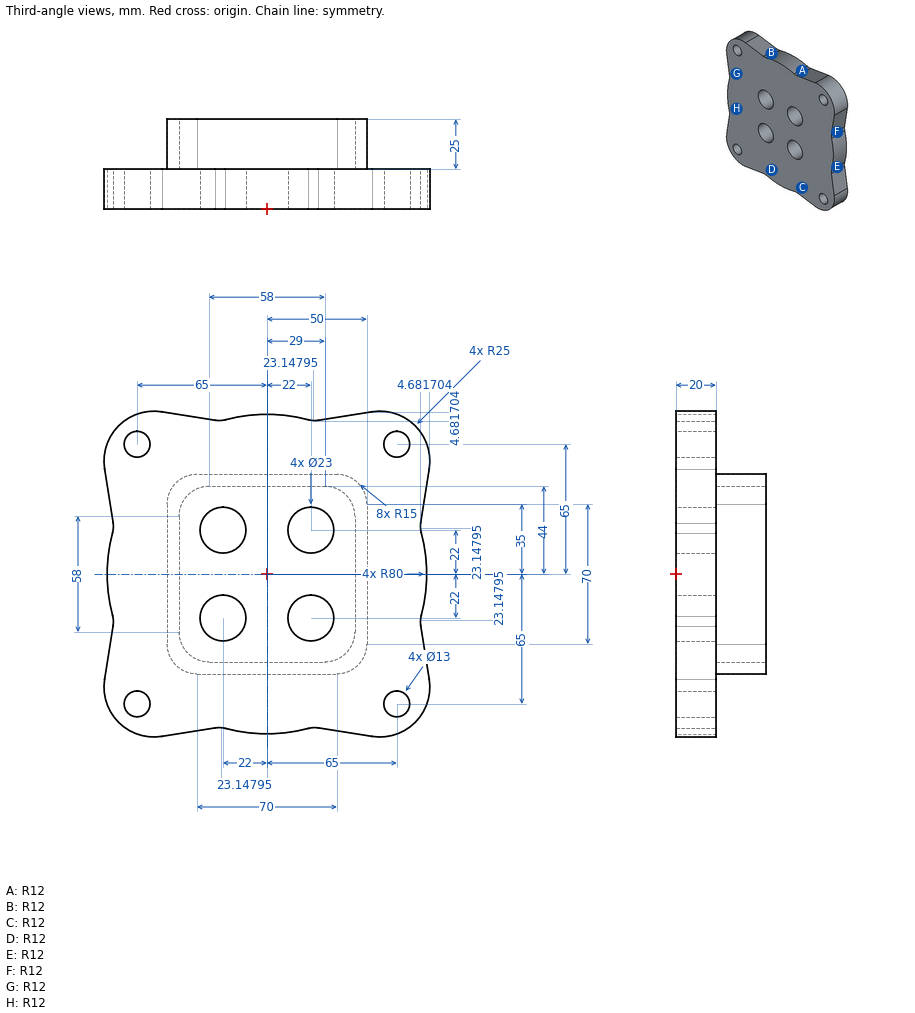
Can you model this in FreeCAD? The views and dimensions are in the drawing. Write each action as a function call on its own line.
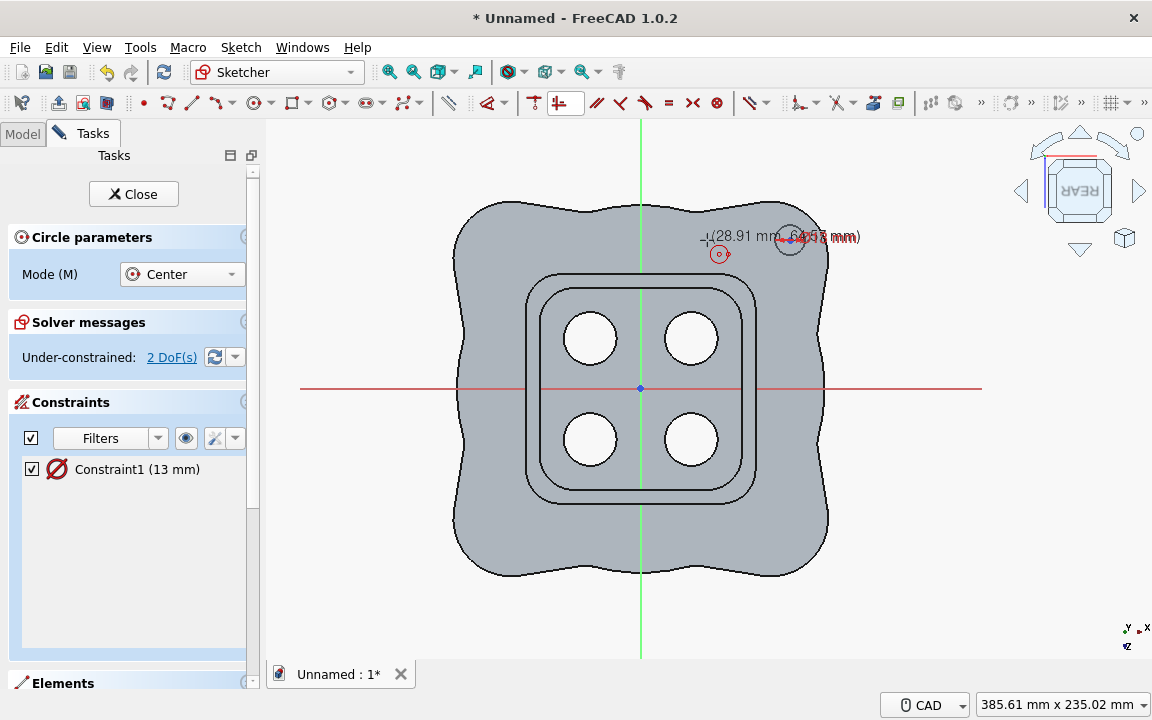
scroll(790, 538, up, 3)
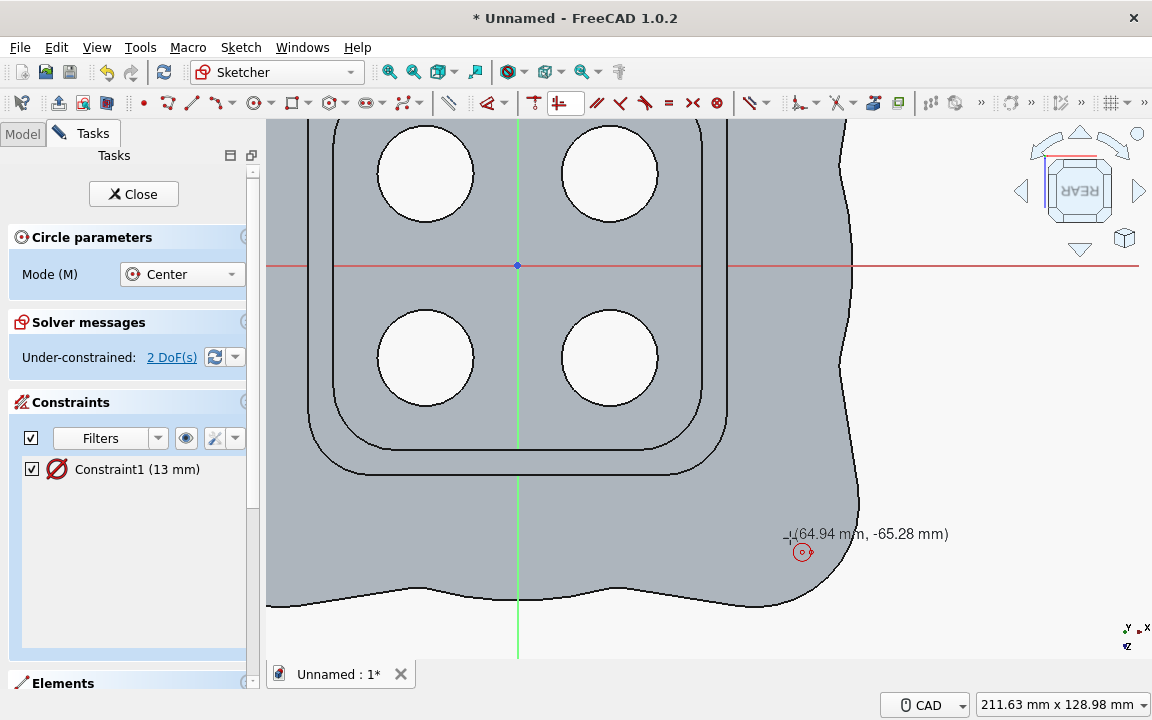
click(790, 538)
move(809, 519)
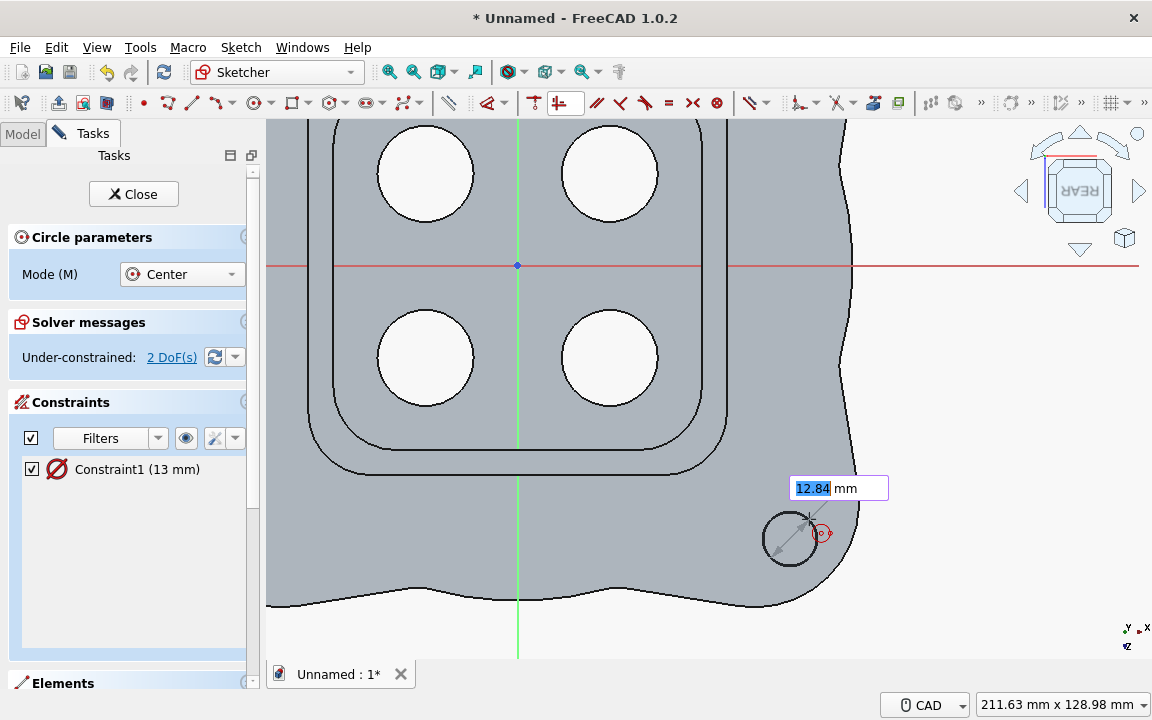
text(13)
key(Return)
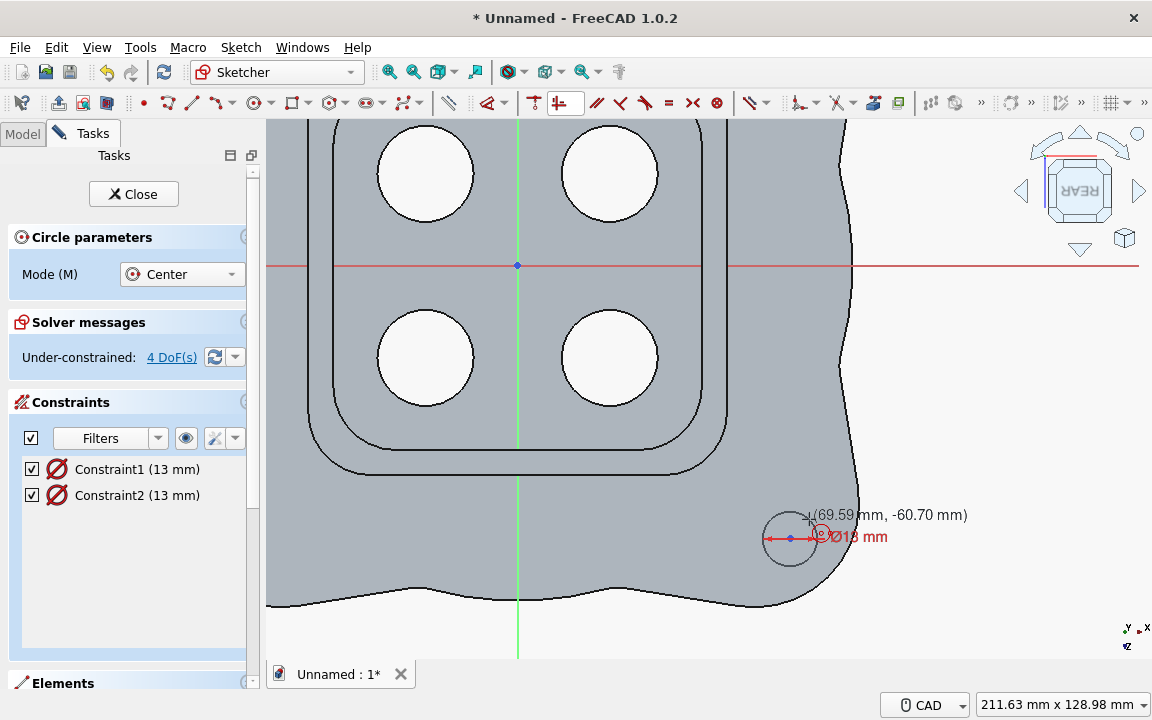
scroll(790, 539, down, 3)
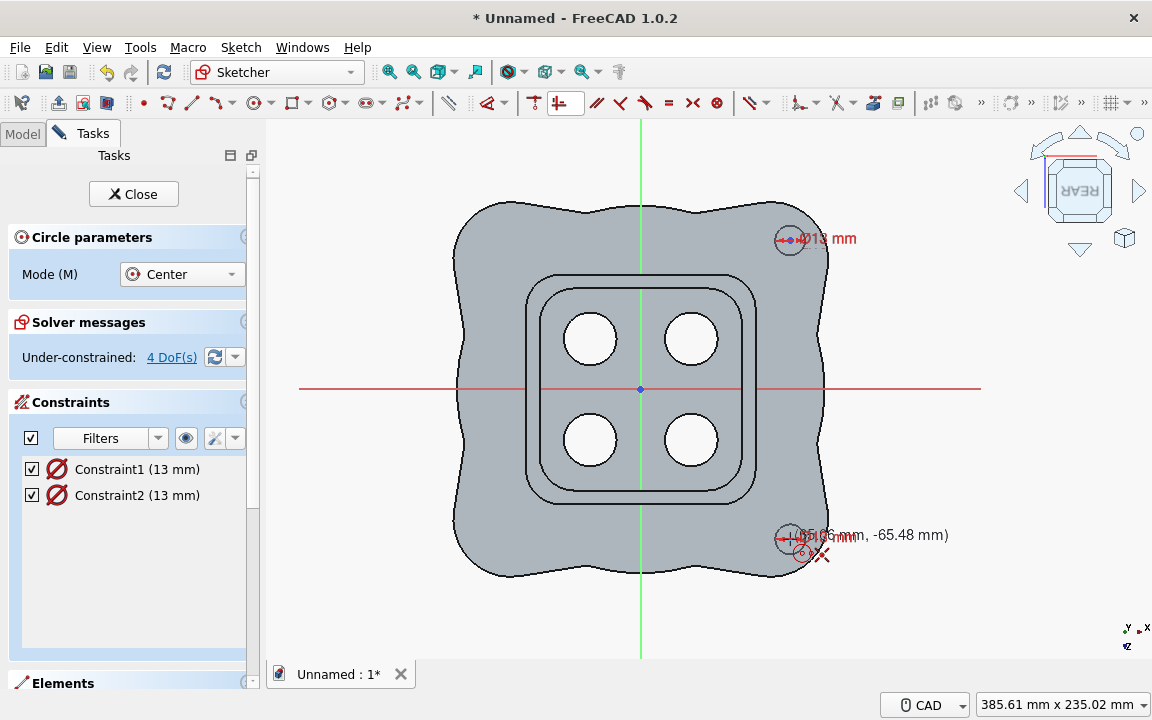
scroll(491, 539, up, 3)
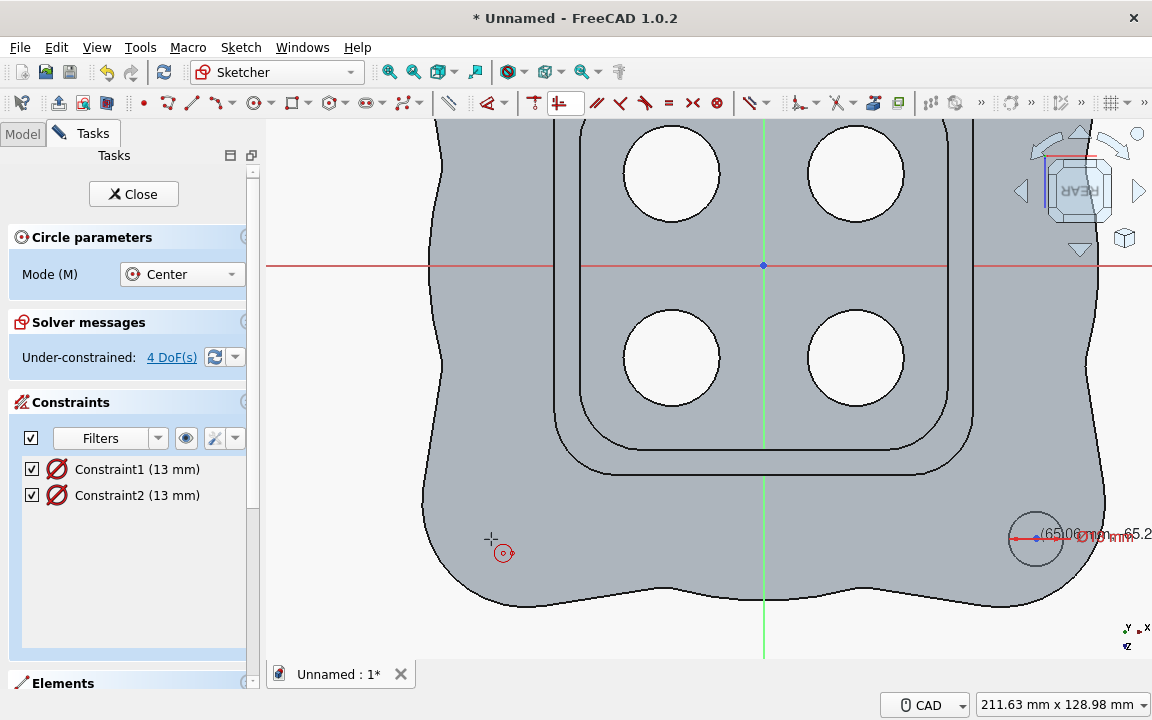
click(492, 538)
move(511, 519)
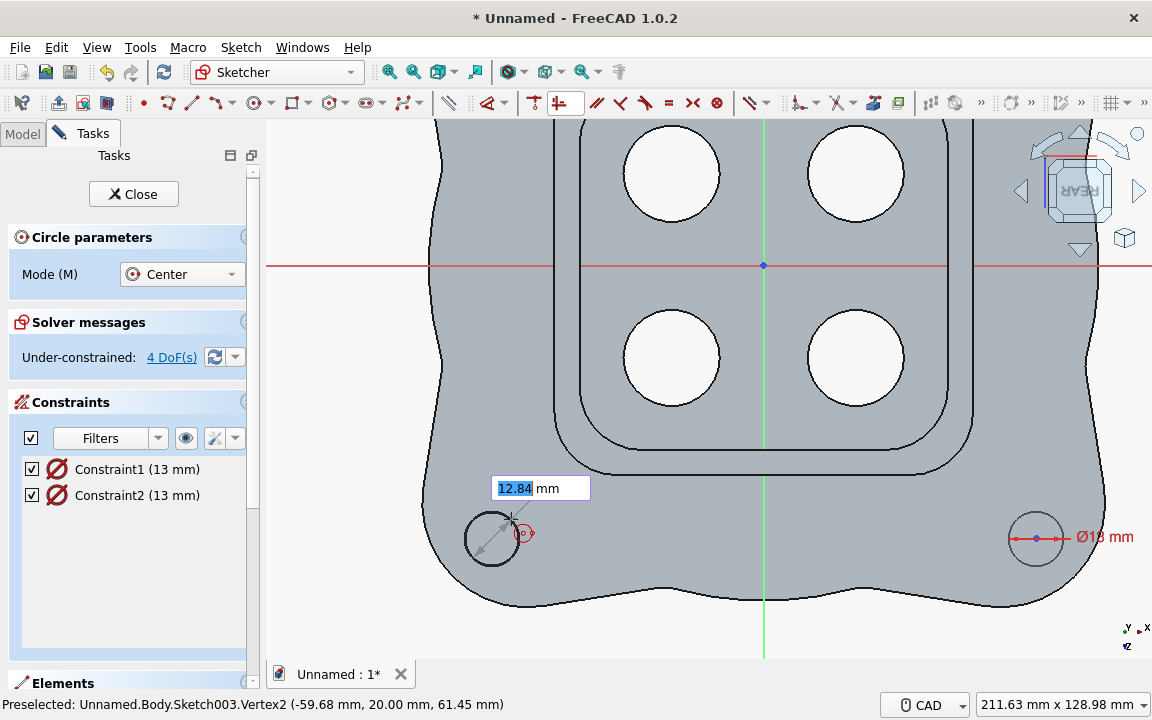
text(13)
key(Return)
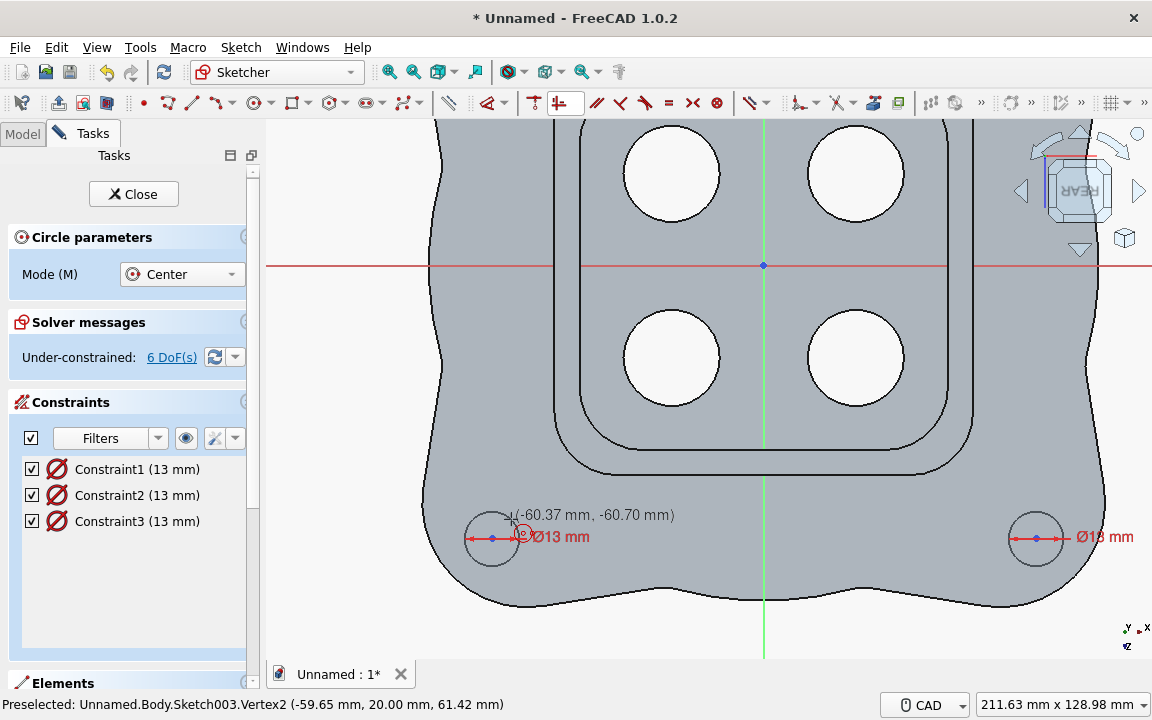
scroll(491, 539, down, 3)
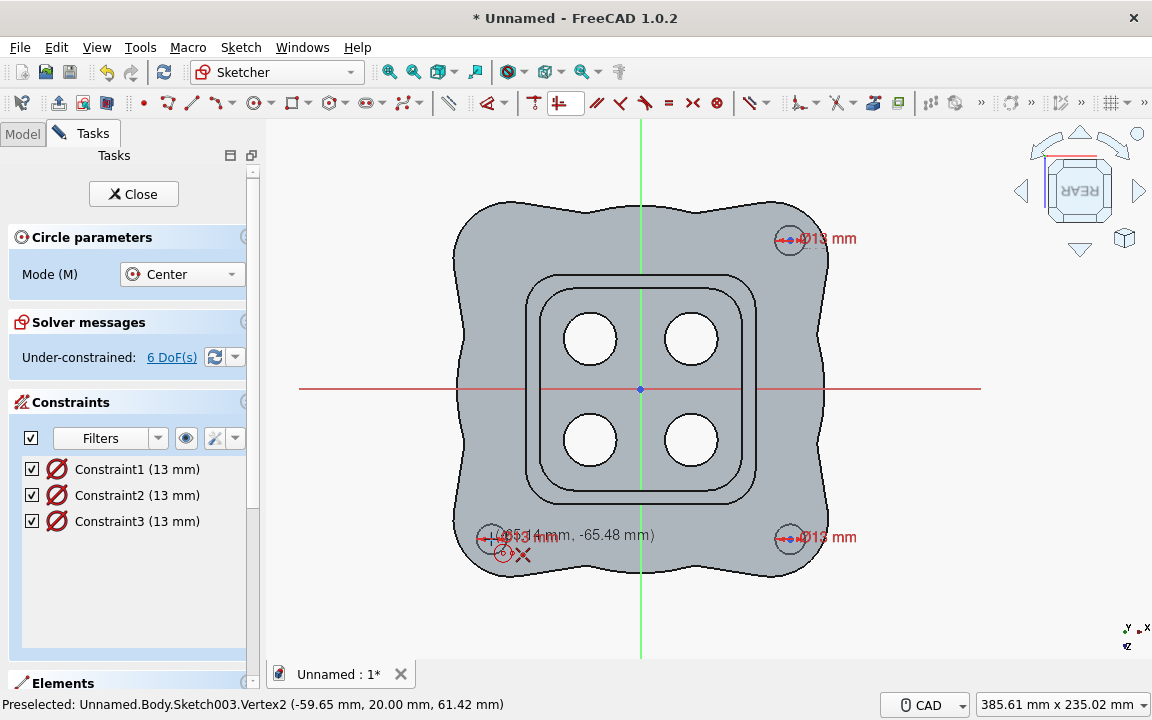
scroll(491, 240, up, 3)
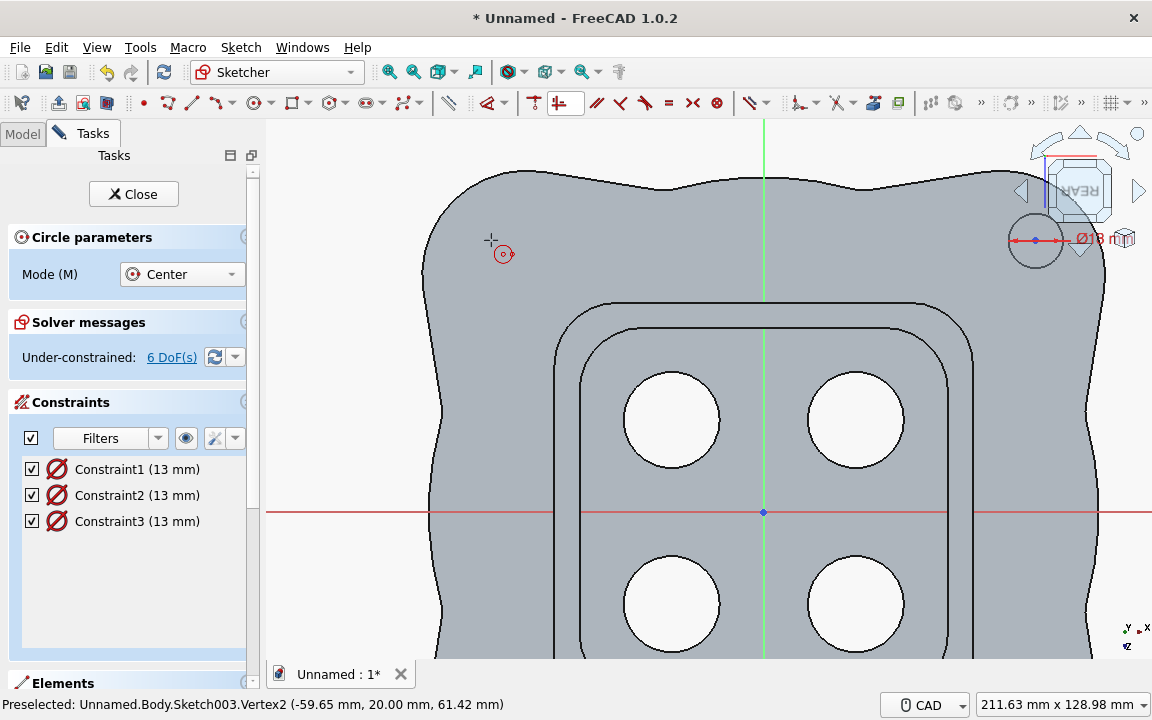
click(492, 240)
move(511, 221)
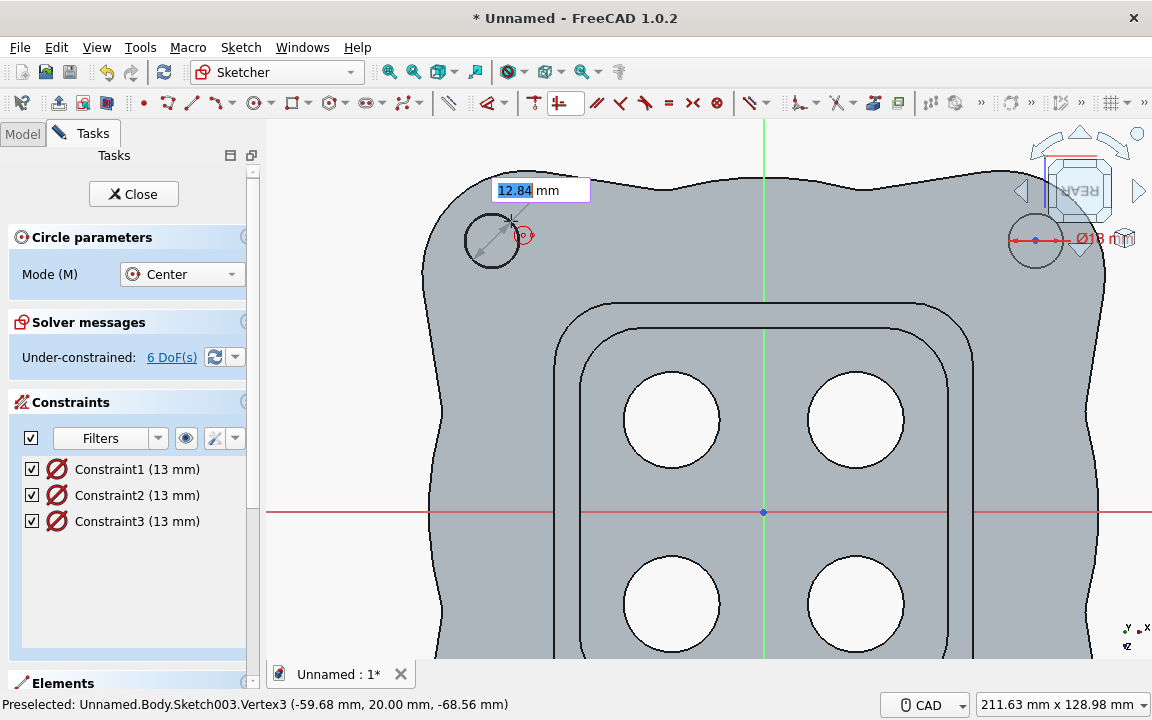
text(13)
key(Return)
key(Escape)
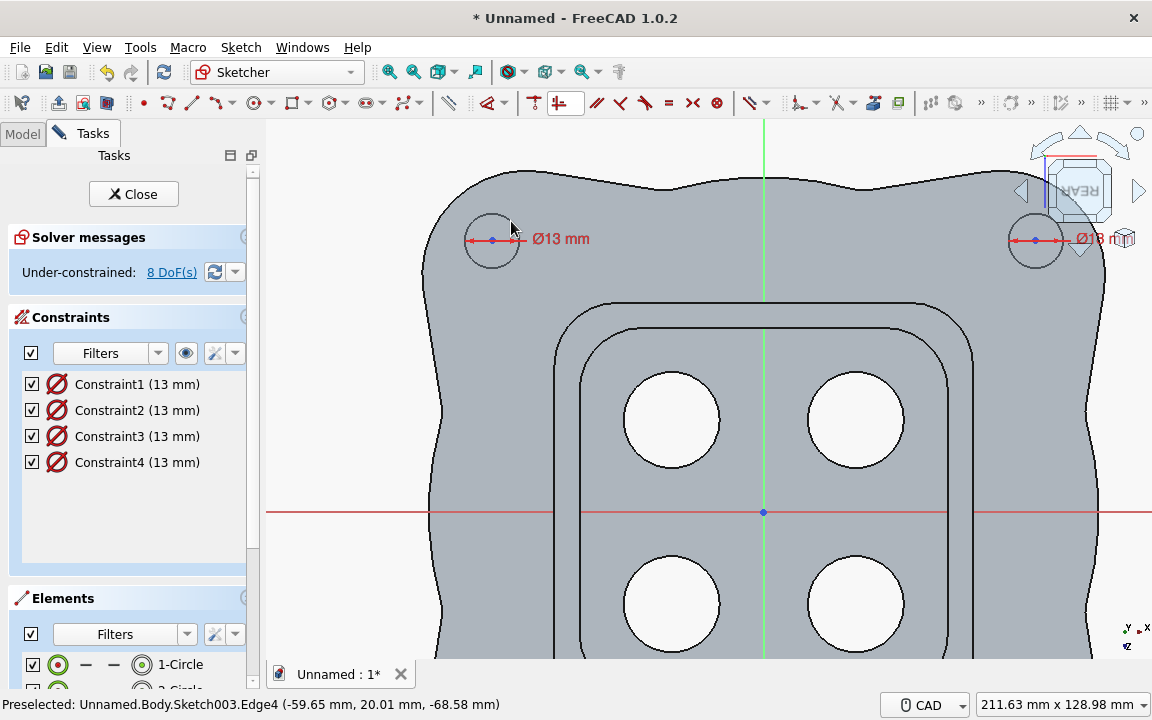
scroll(491, 239, down, 3)